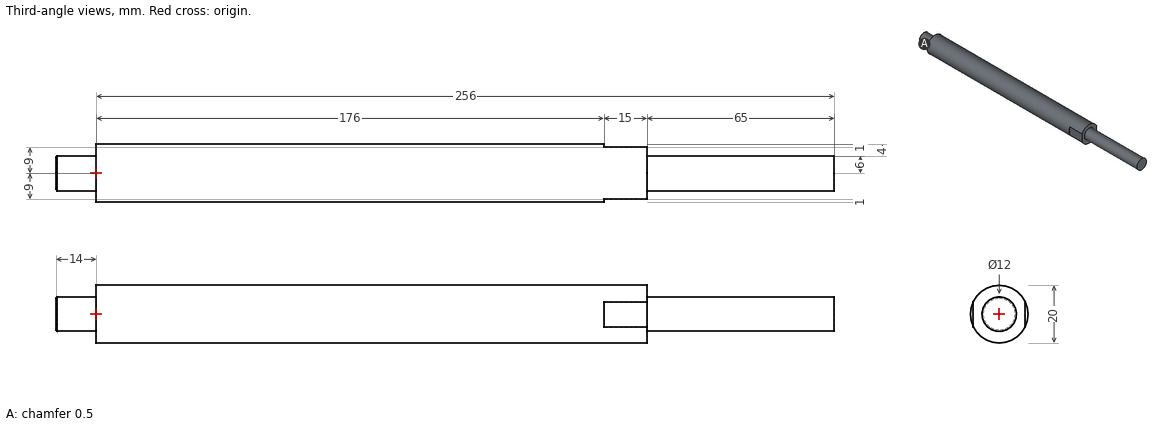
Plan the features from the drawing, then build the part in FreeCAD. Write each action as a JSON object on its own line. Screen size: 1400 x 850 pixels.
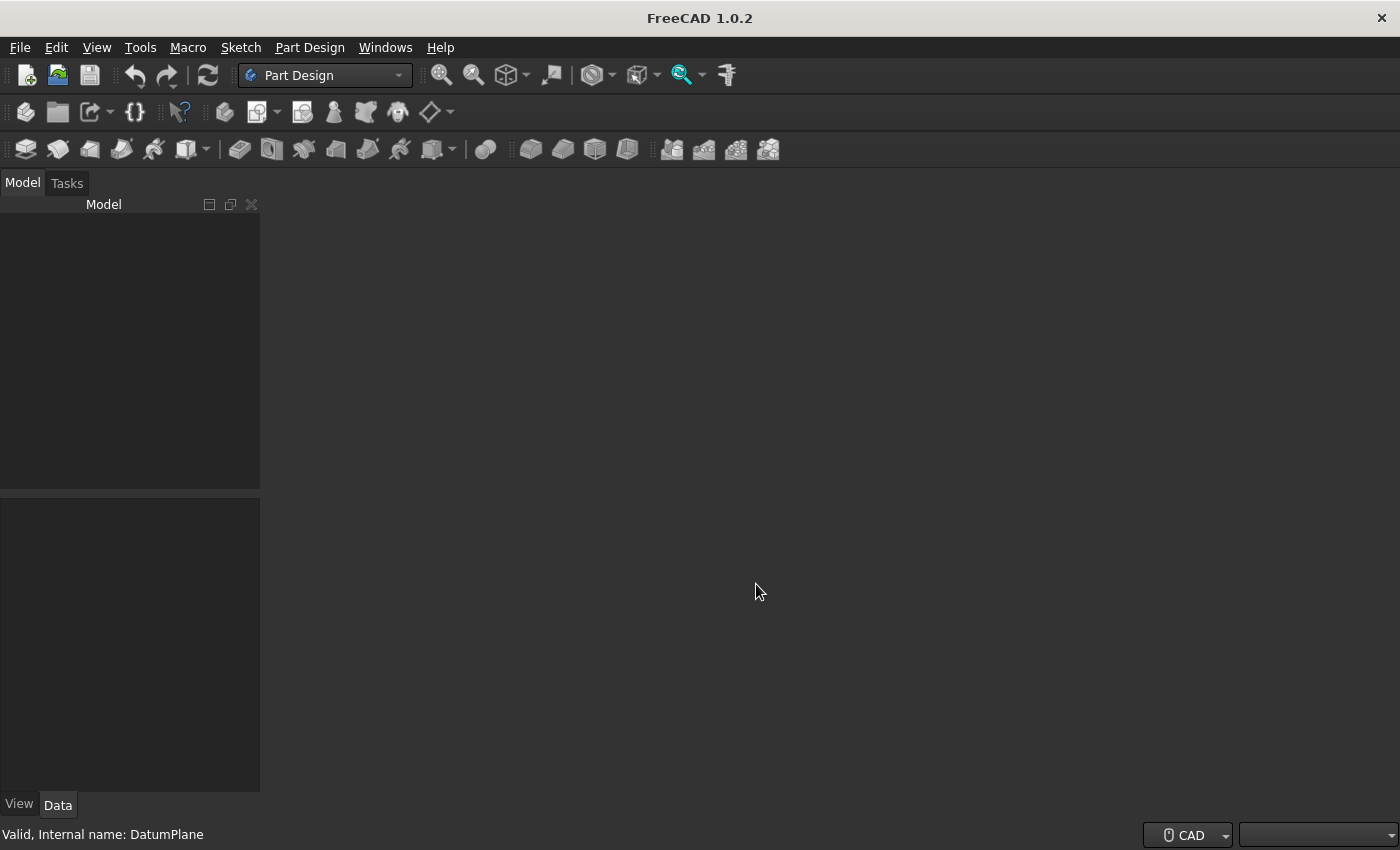
{"action": "key", "text": "ctrl+n"}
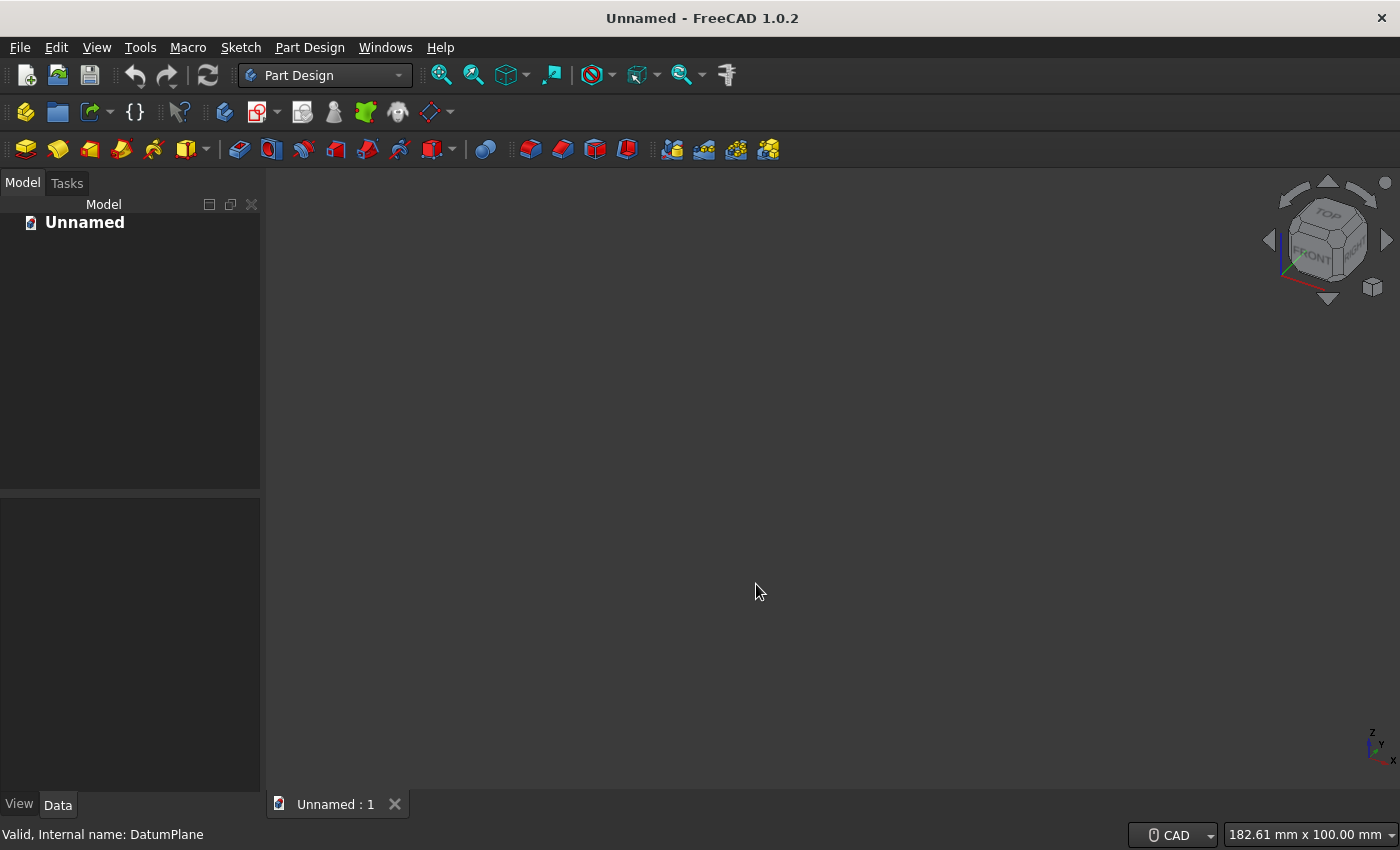
{"action": "left_click", "coordinate": [258, 112]}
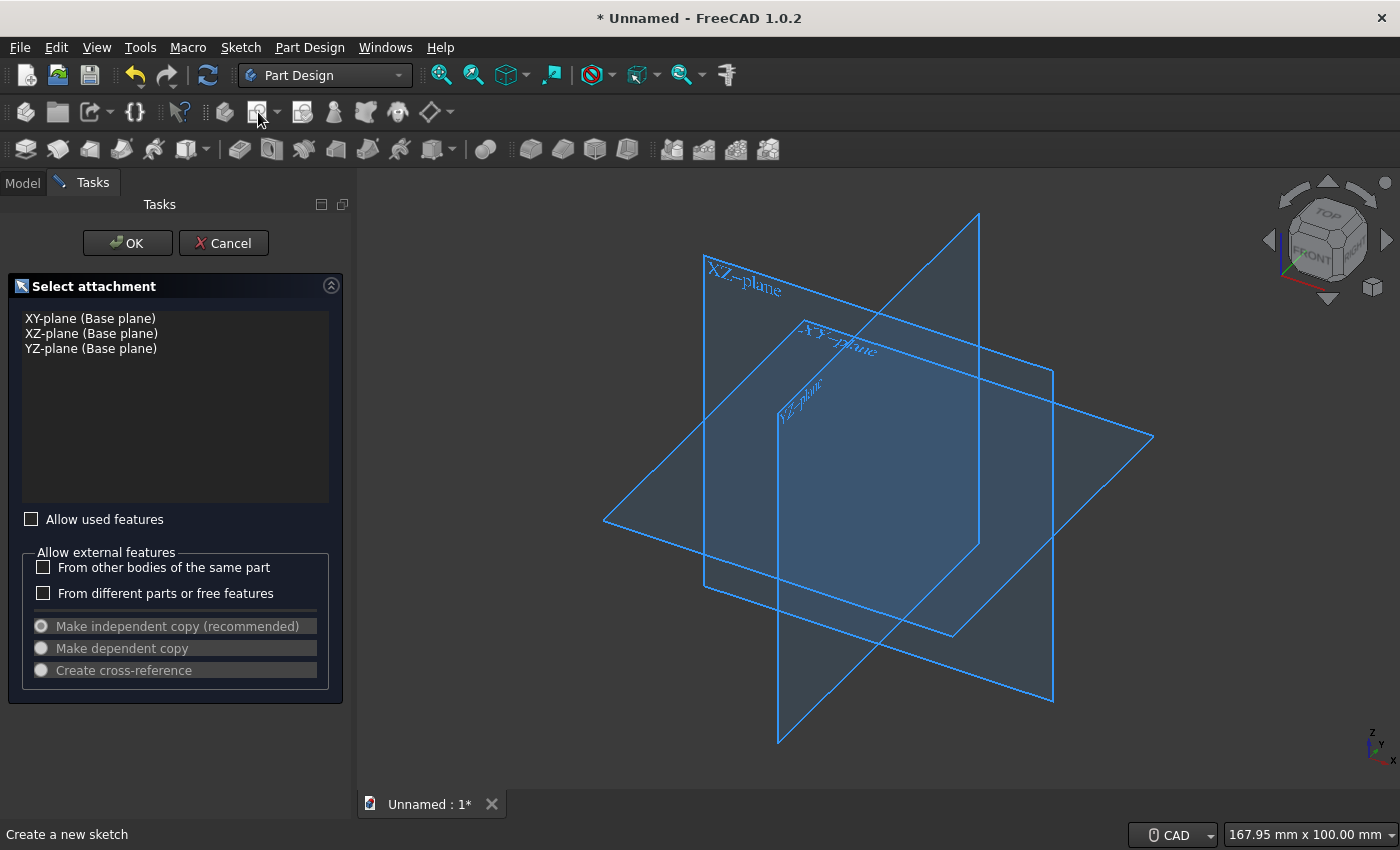
{"action": "left_click", "coordinate": [82, 318]}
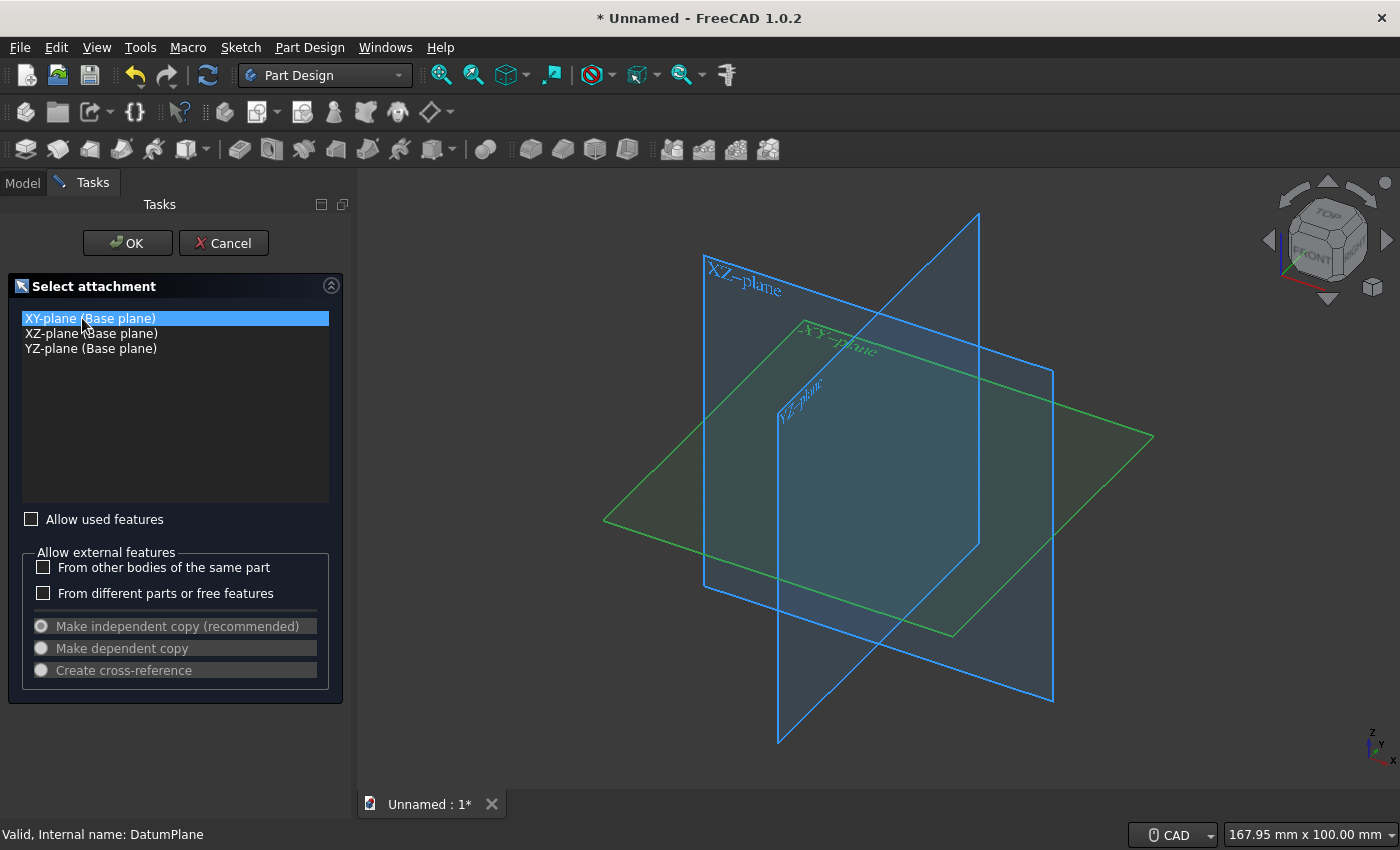
{"action": "left_click", "coordinate": [128, 243]}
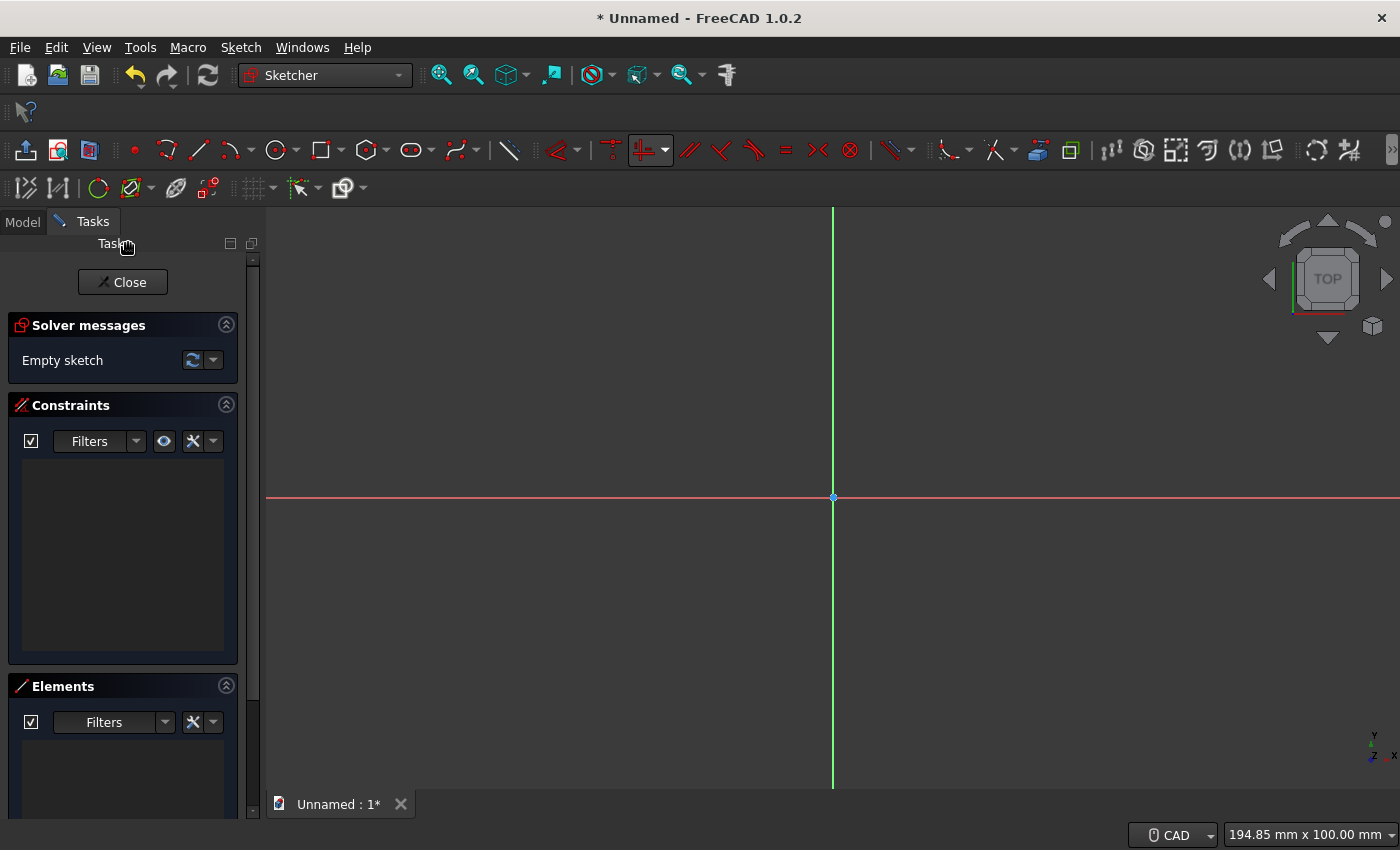
{"action": "scroll", "coordinate": [294, 522], "scroll_direction": "down", "scroll_amount": 4}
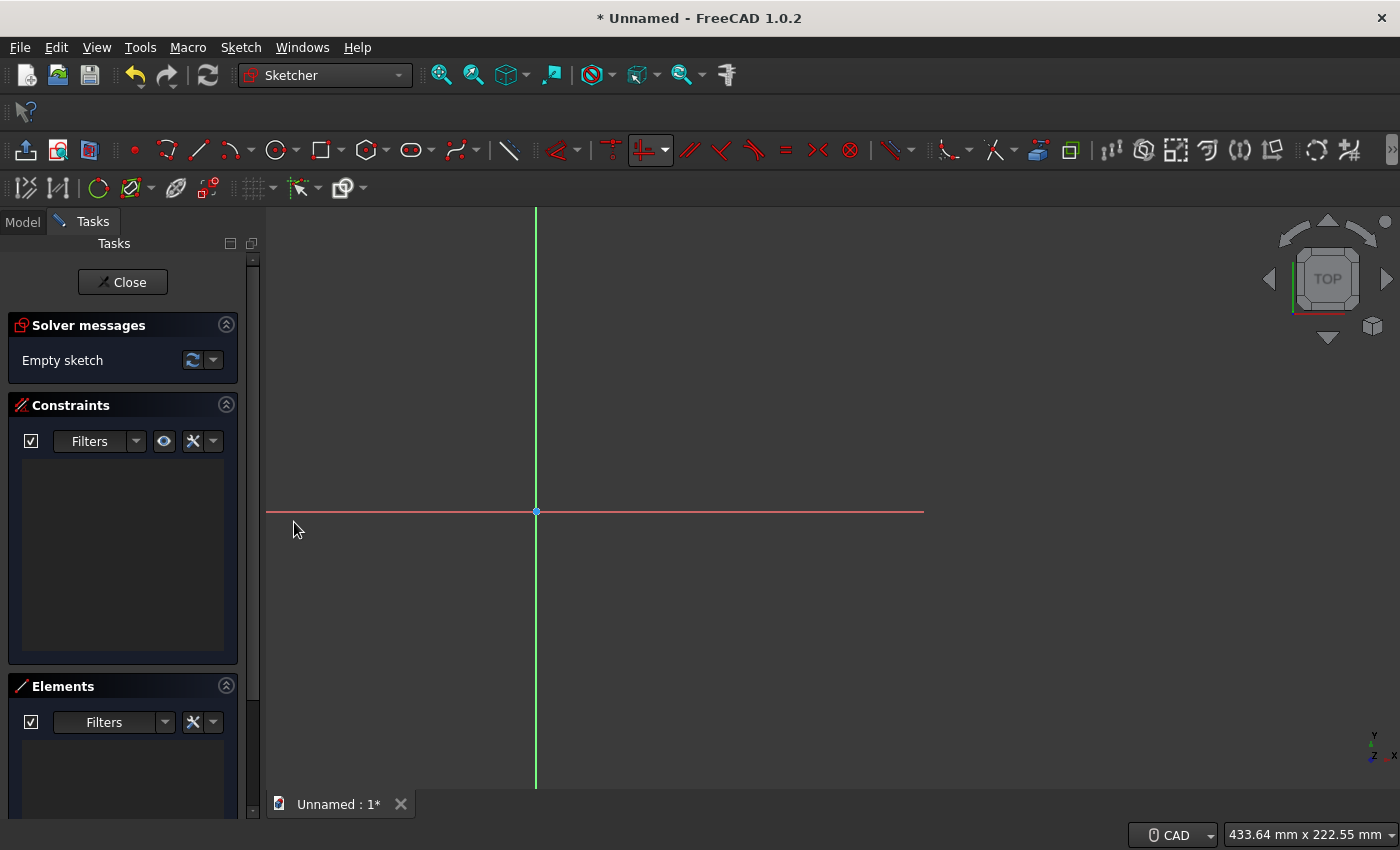
{"action": "left_click", "coordinate": [168, 150]}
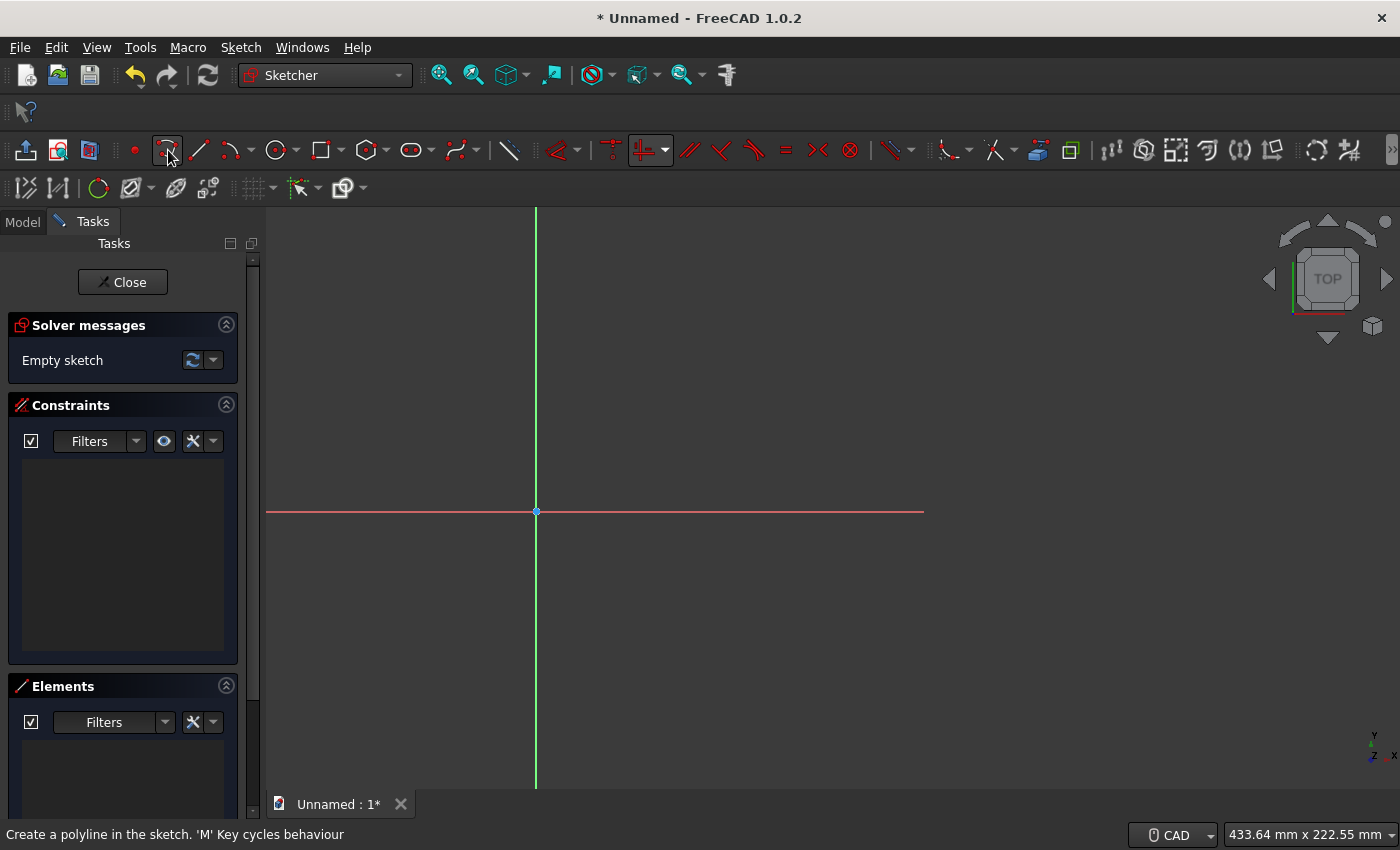
{"action": "left_click", "coordinate": [536, 512]}
{"action": "left_click", "coordinate": [1206, 503]}
{"action": "left_click", "coordinate": [1206, 496]}
{"action": "left_click", "coordinate": [1036, 496]}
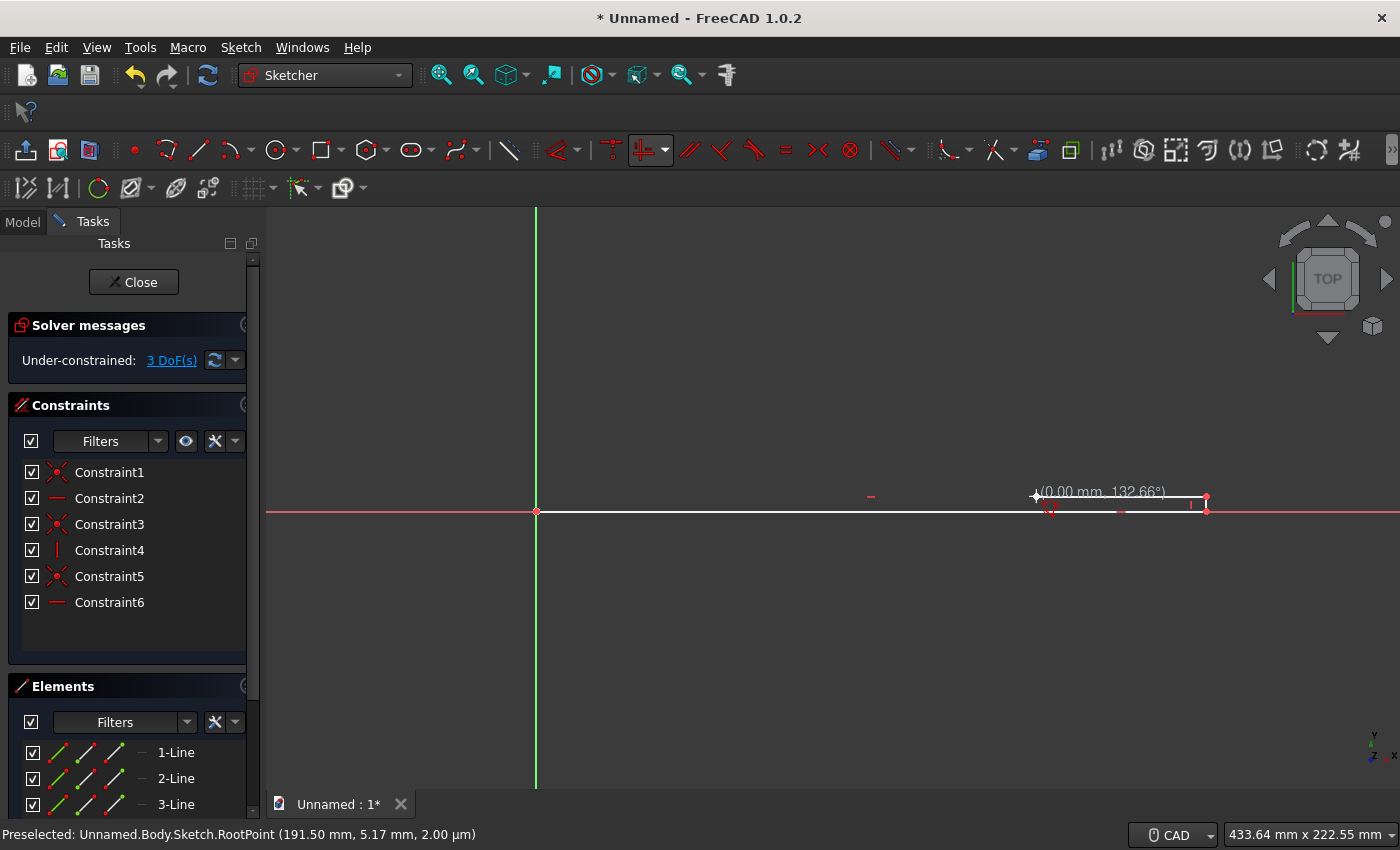
{"action": "scroll", "coordinate": [1036, 485], "scroll_direction": "up", "scroll_amount": 3}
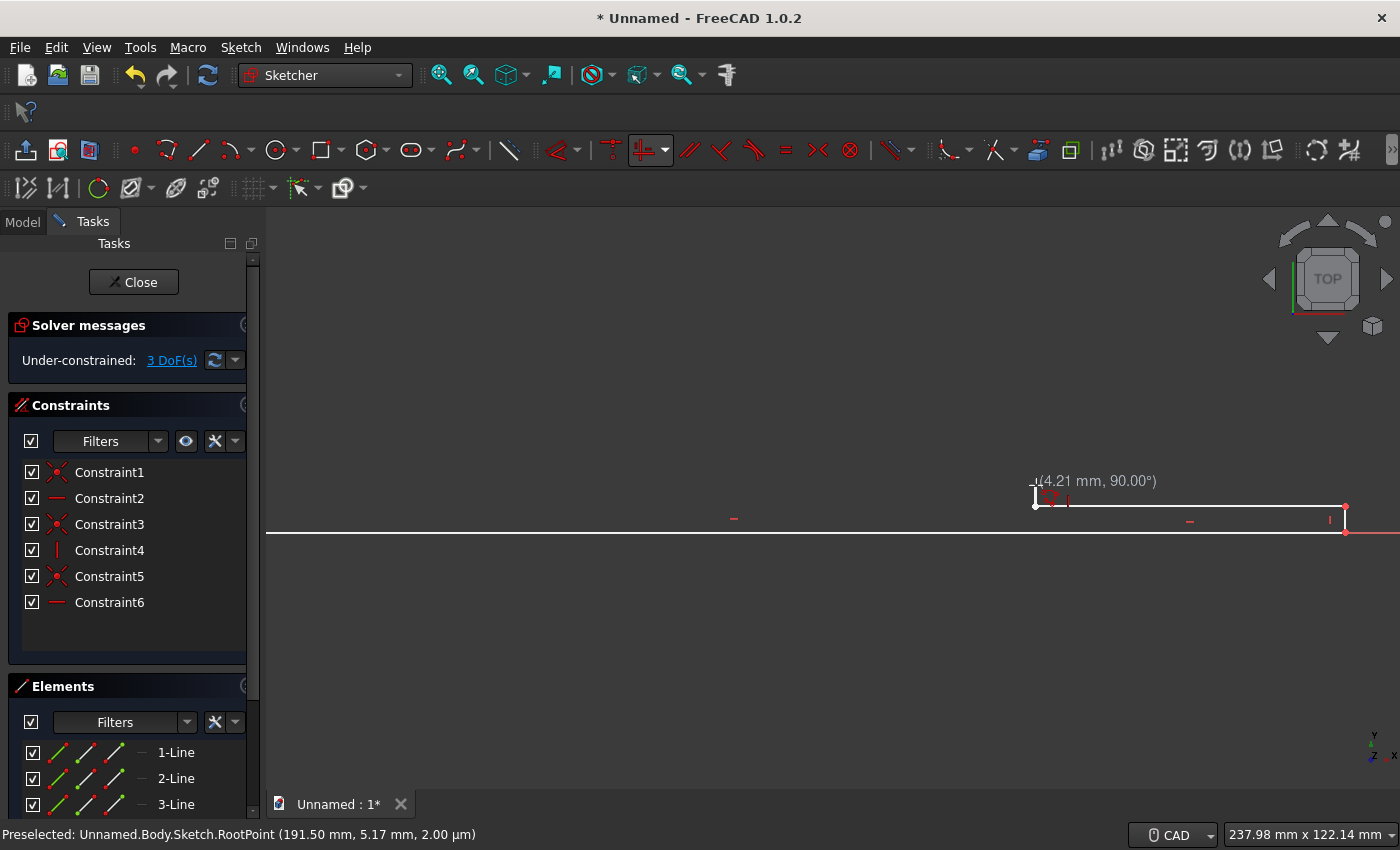
{"action": "left_click", "coordinate": [1035, 485]}